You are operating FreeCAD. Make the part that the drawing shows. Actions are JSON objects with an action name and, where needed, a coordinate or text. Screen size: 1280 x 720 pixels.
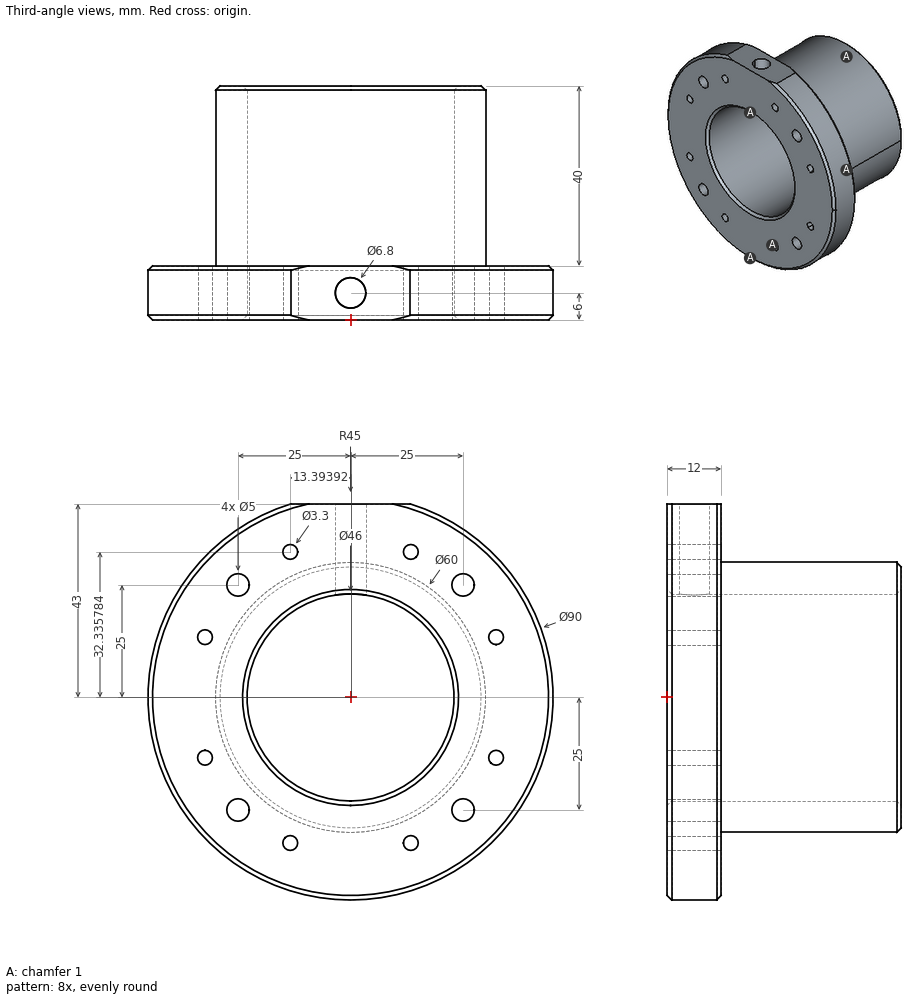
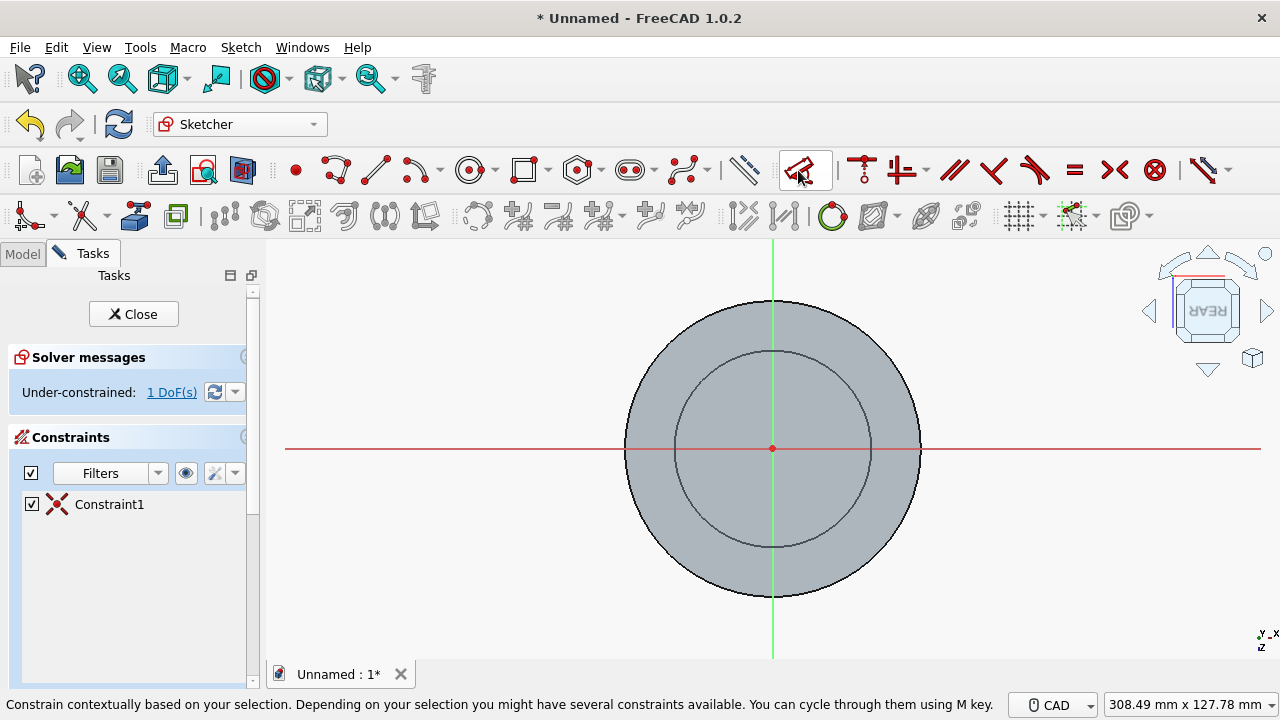
{"action": "left_click", "coordinate": [842, 379]}
{"action": "left_click", "coordinate": [864, 356]}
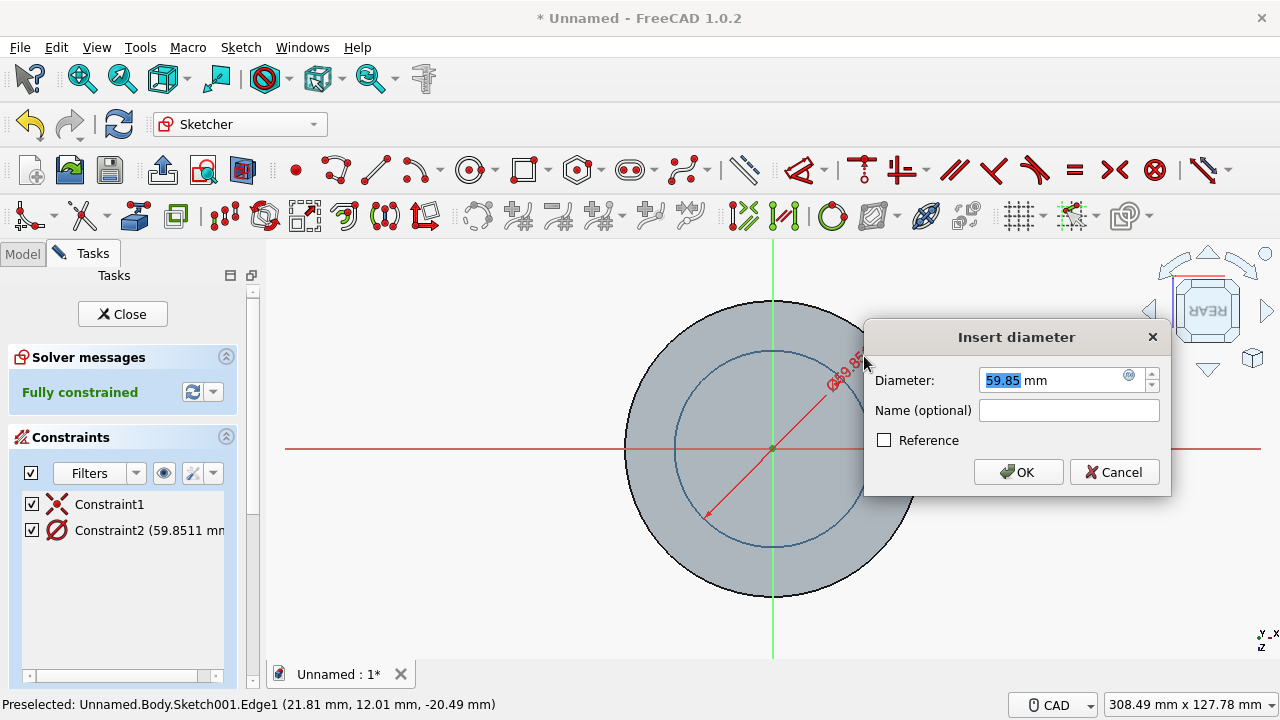
{"action": "type", "text": "60"}
{"action": "key", "text": "Return"}
{"action": "key", "text": "Escape"}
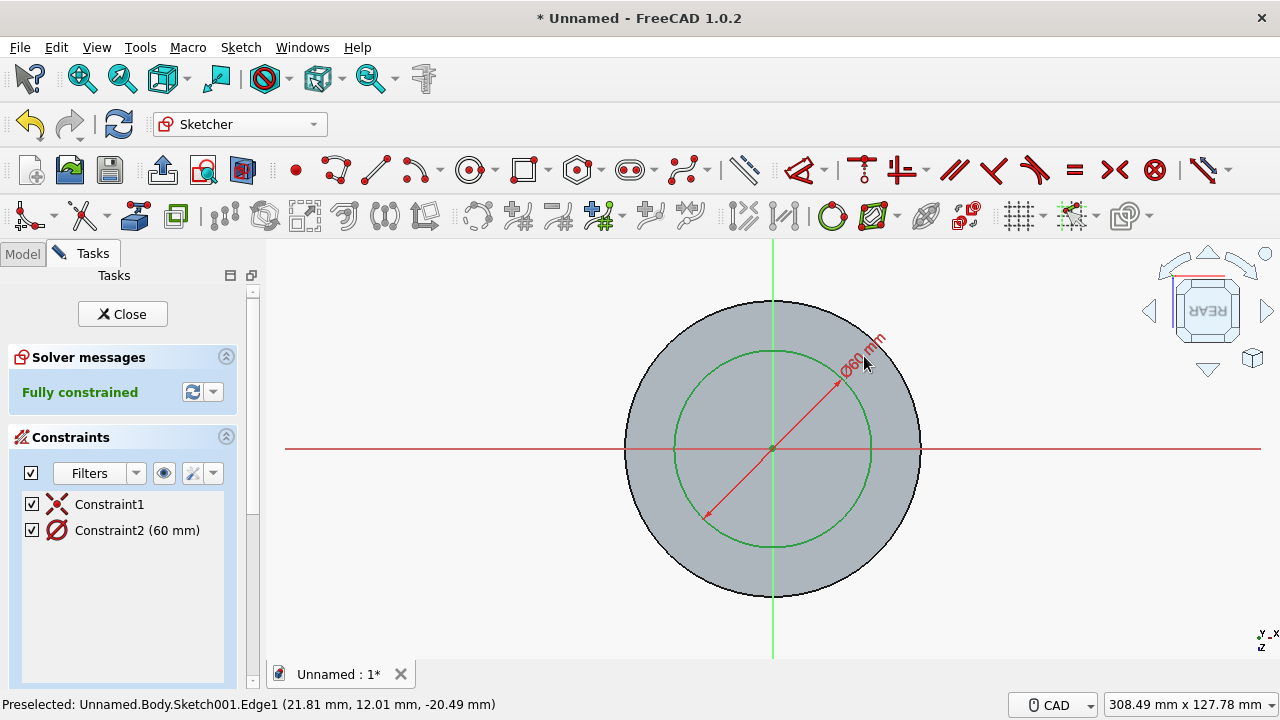
{"action": "left_click", "coordinate": [123, 314]}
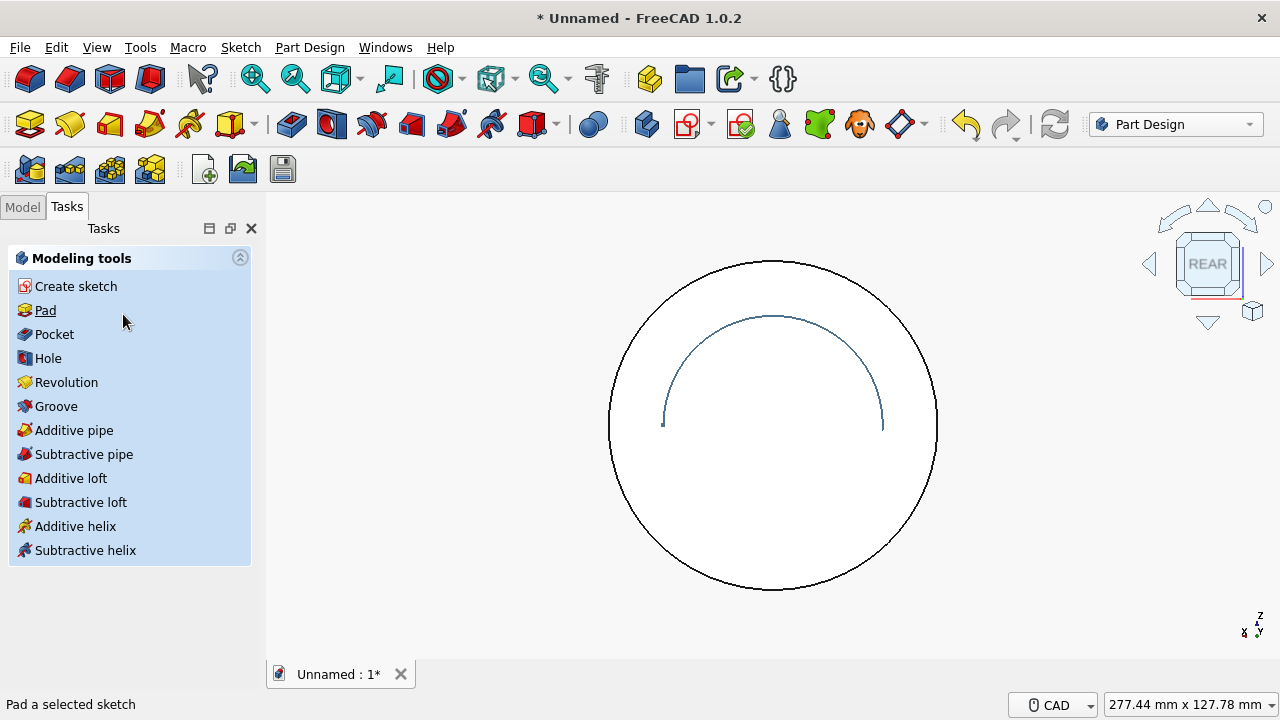
{"action": "left_click", "coordinate": [30, 124]}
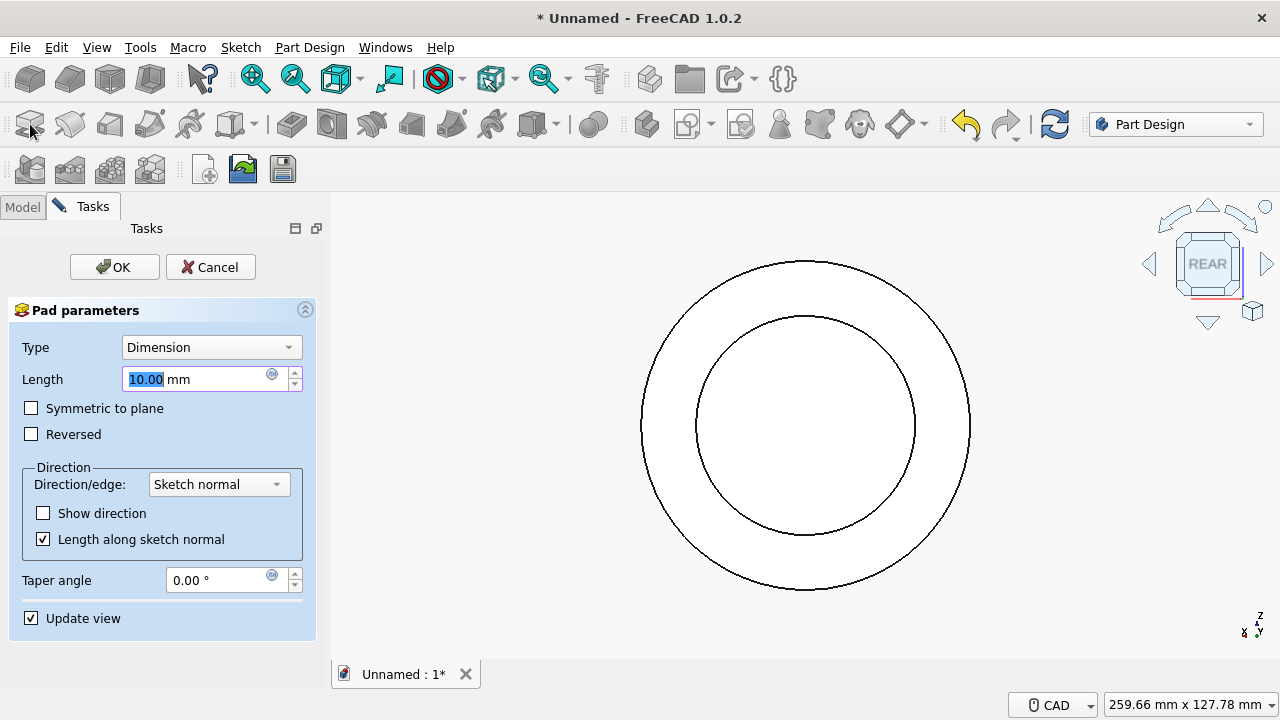
{"action": "type", "text": "40"}
{"action": "key", "text": "Tab"}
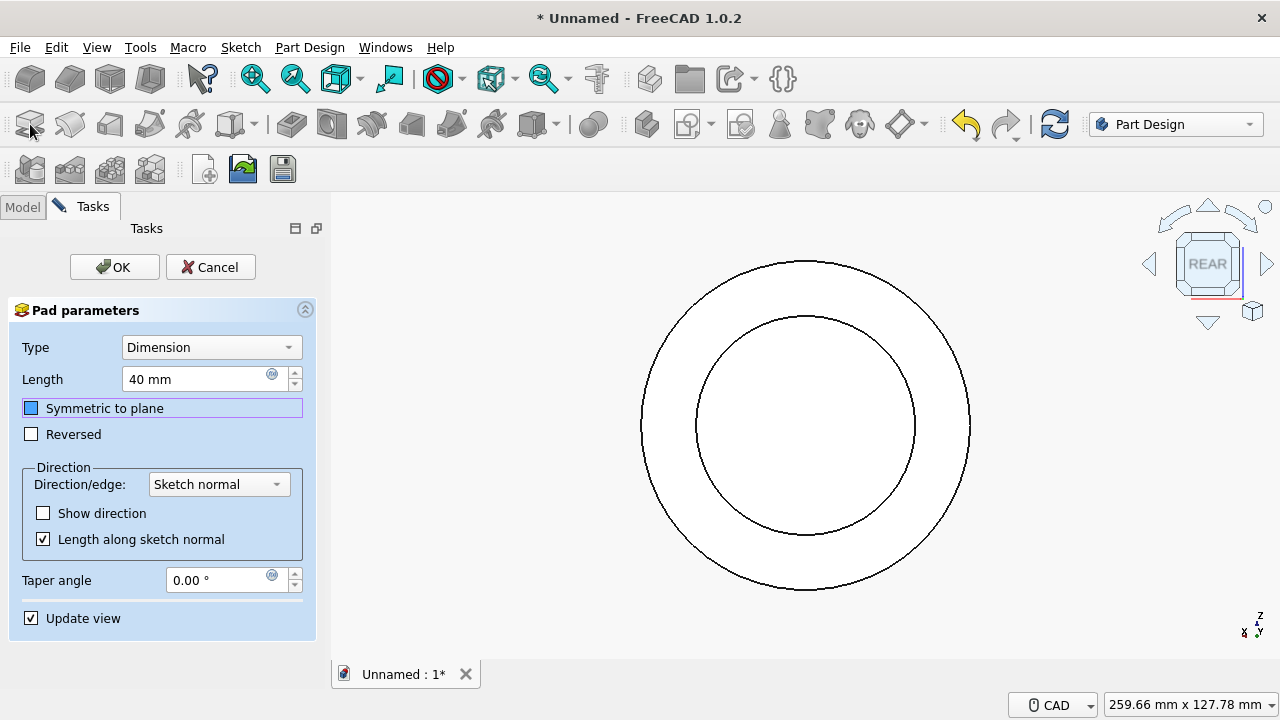
{"action": "left_click", "coordinate": [115, 267]}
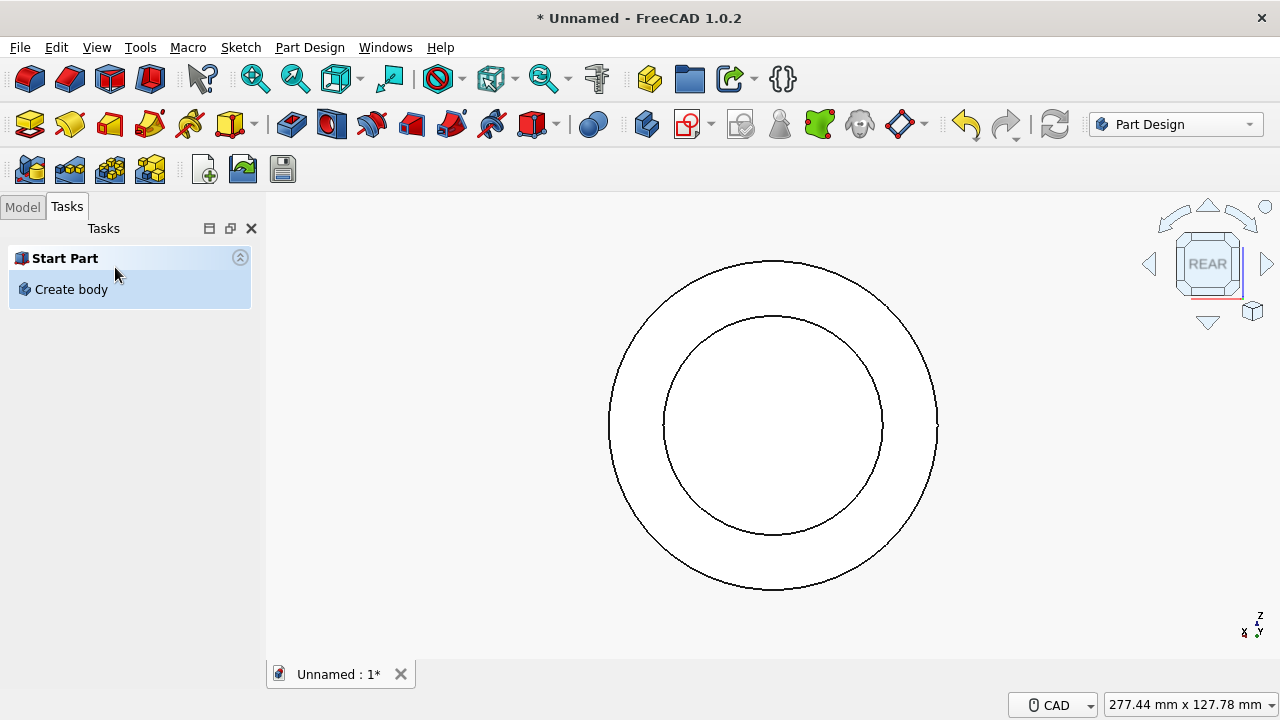
{"action": "key", "text": "0"}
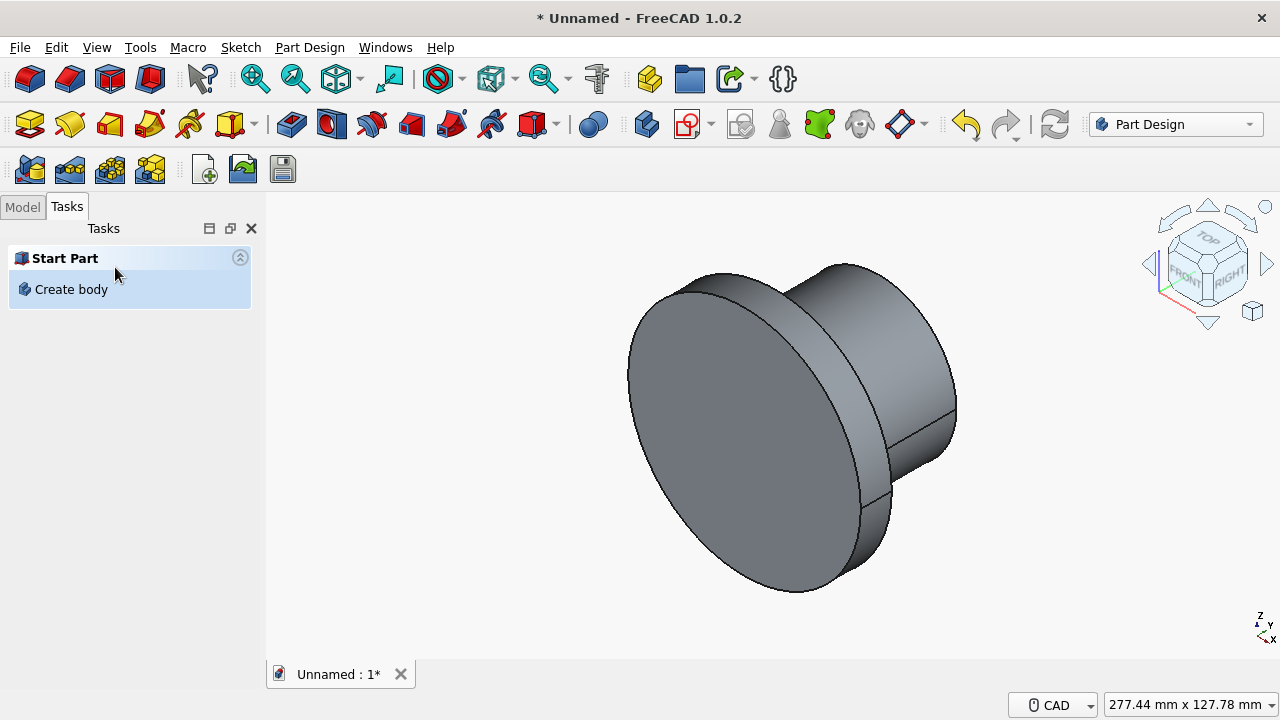
{"action": "key", "text": "v f"}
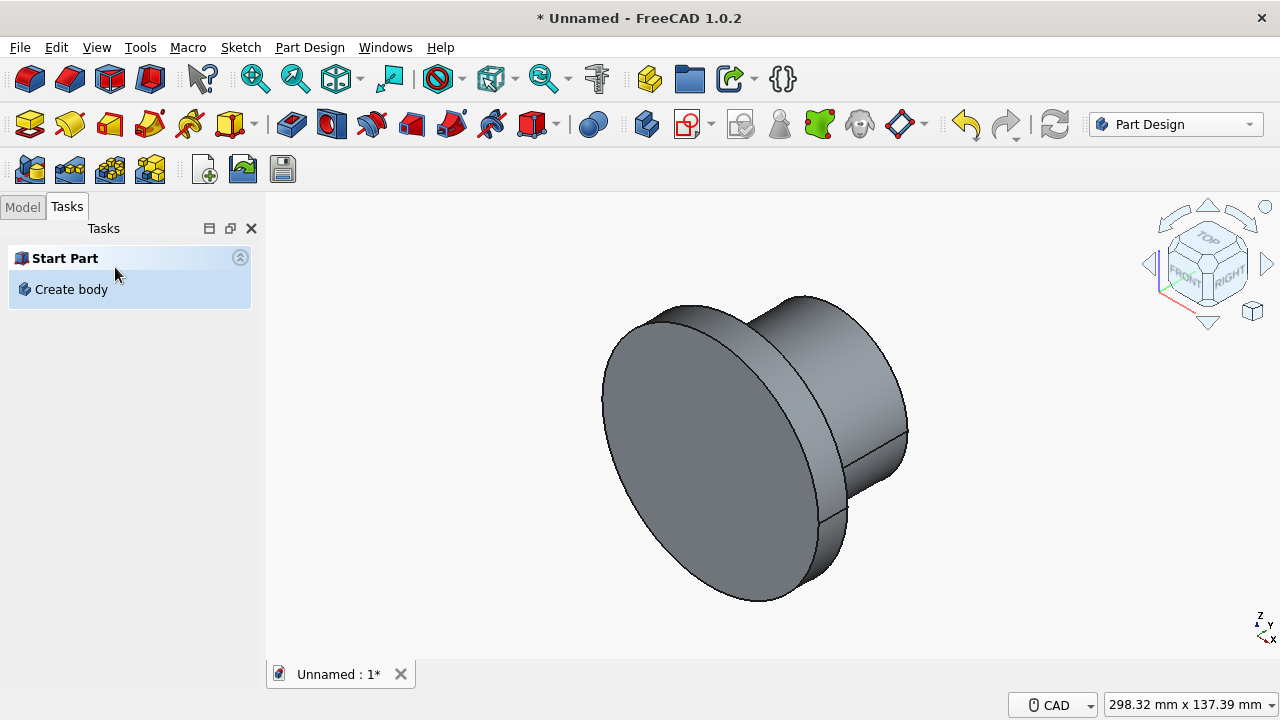
{"action": "left_click", "coordinate": [711, 461]}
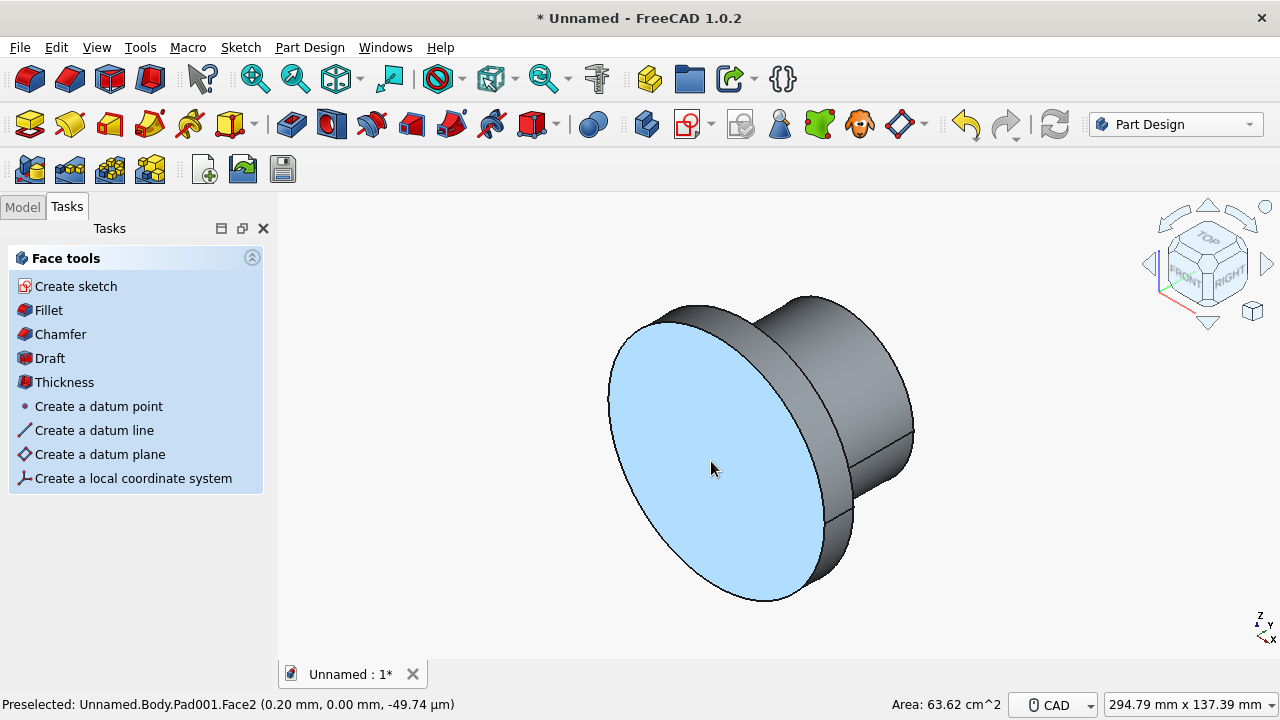
{"action": "left_click", "coordinate": [688, 124]}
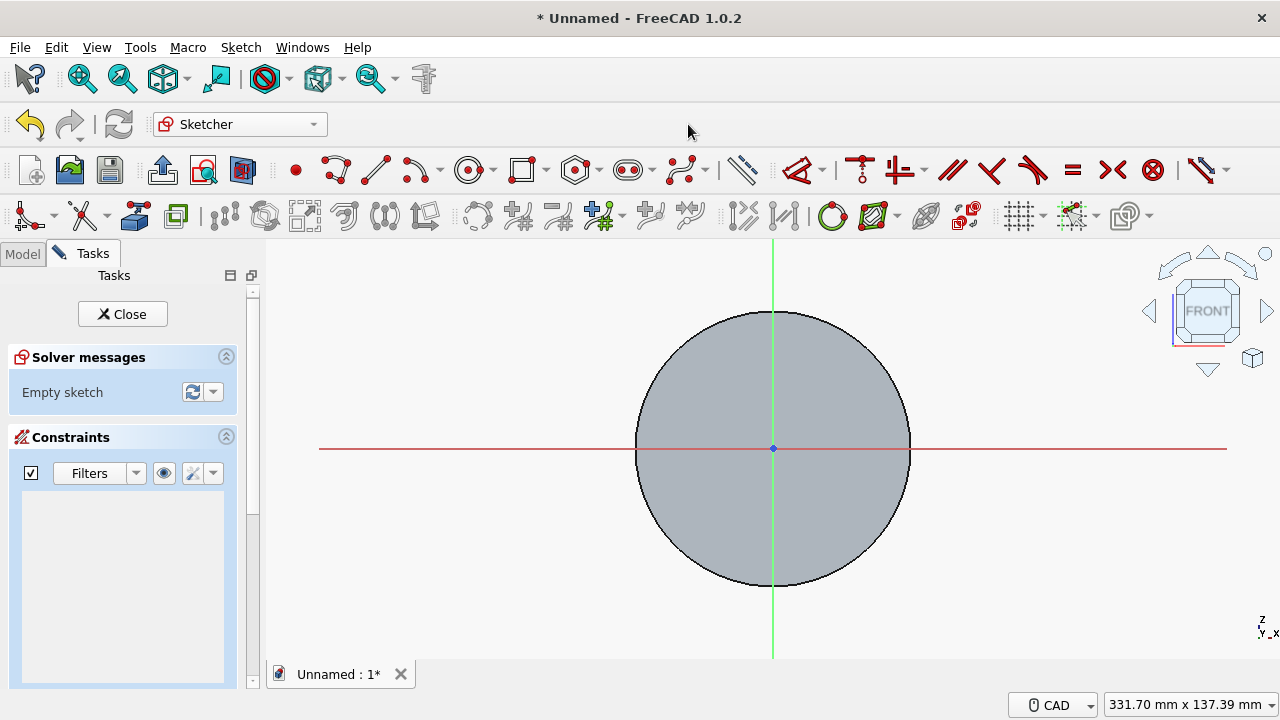
{"action": "scroll", "coordinate": [856, 449], "scroll_direction": "up", "scroll_amount": 3}